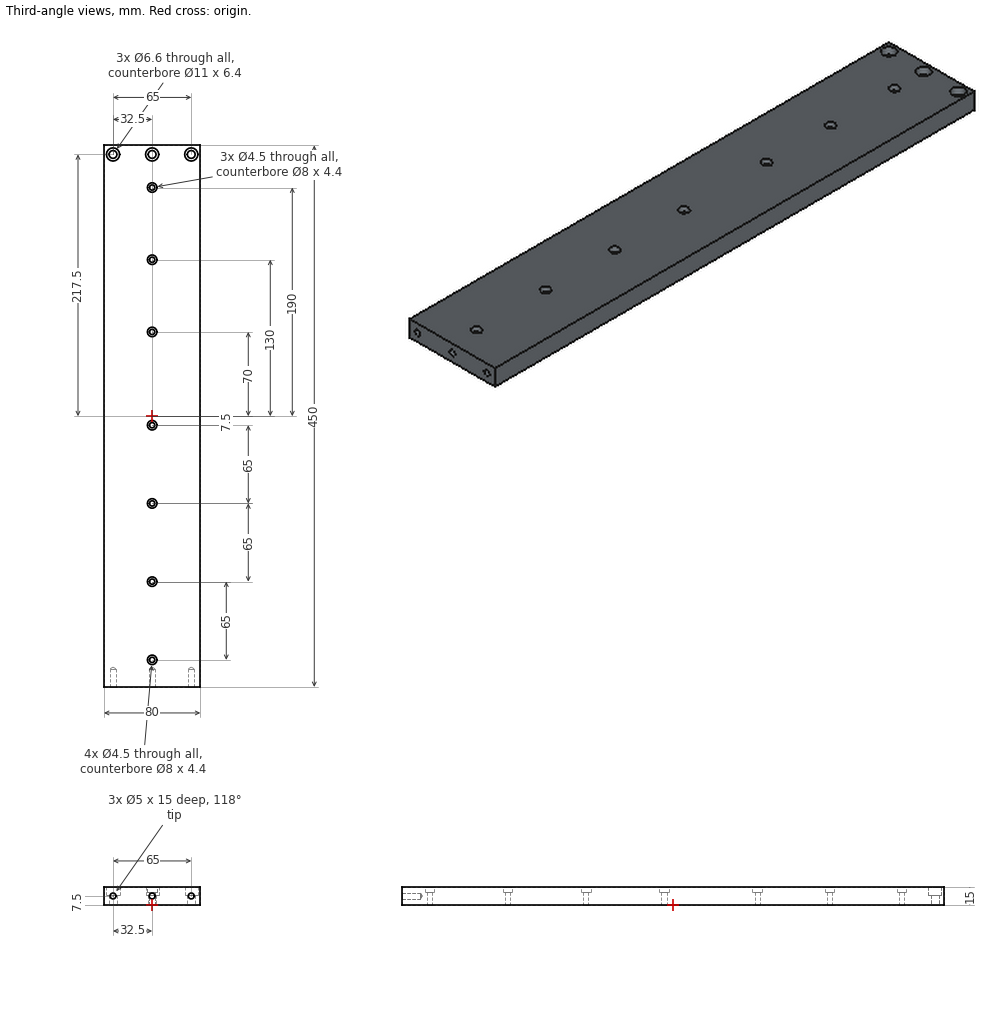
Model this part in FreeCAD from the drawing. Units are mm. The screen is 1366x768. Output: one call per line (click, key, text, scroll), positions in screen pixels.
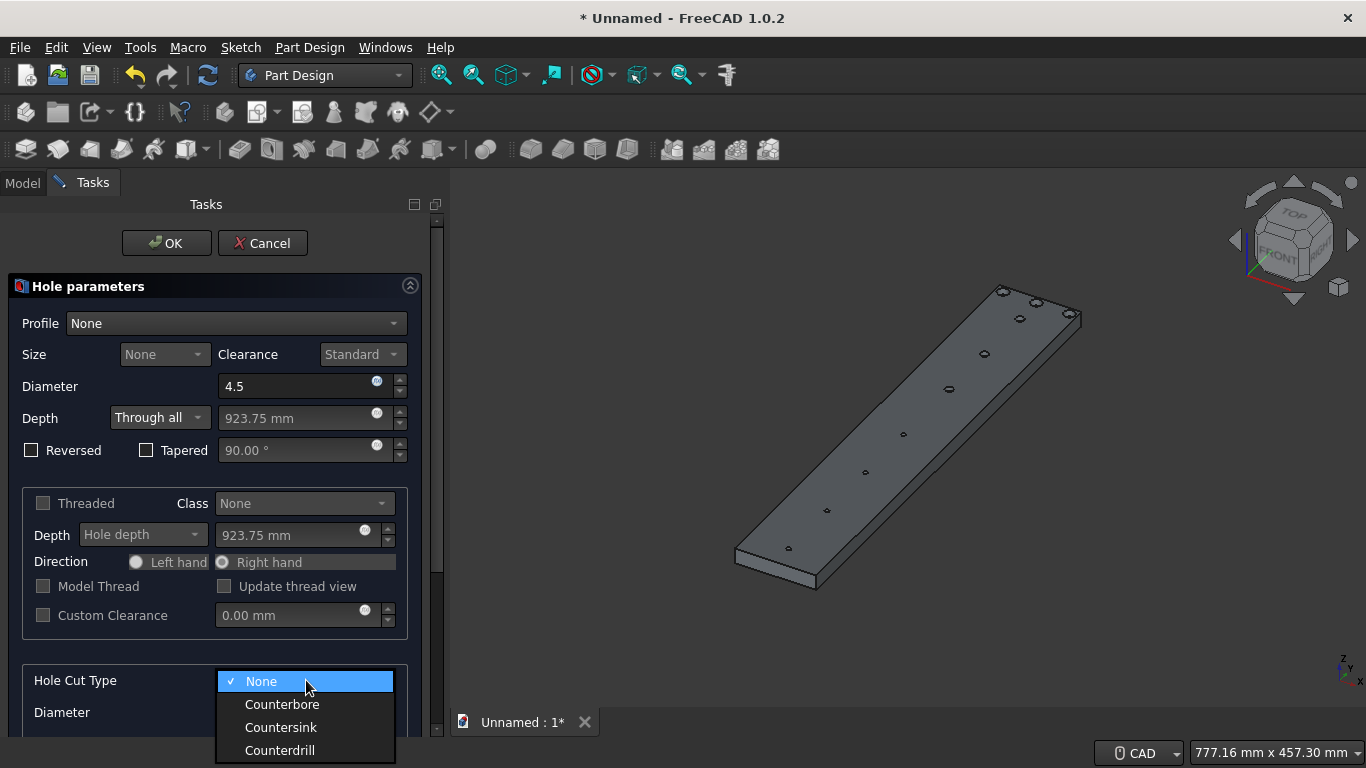
click(304, 704)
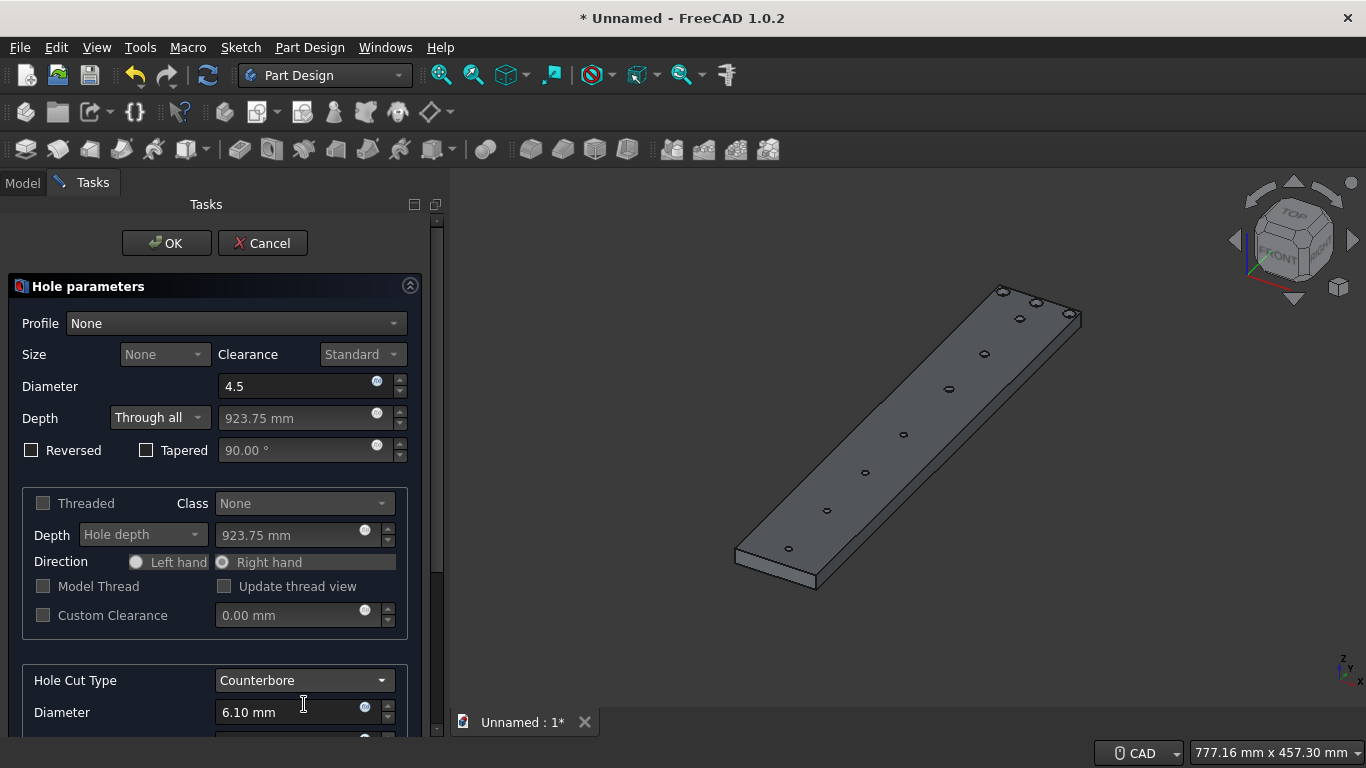
triple_click(298, 712)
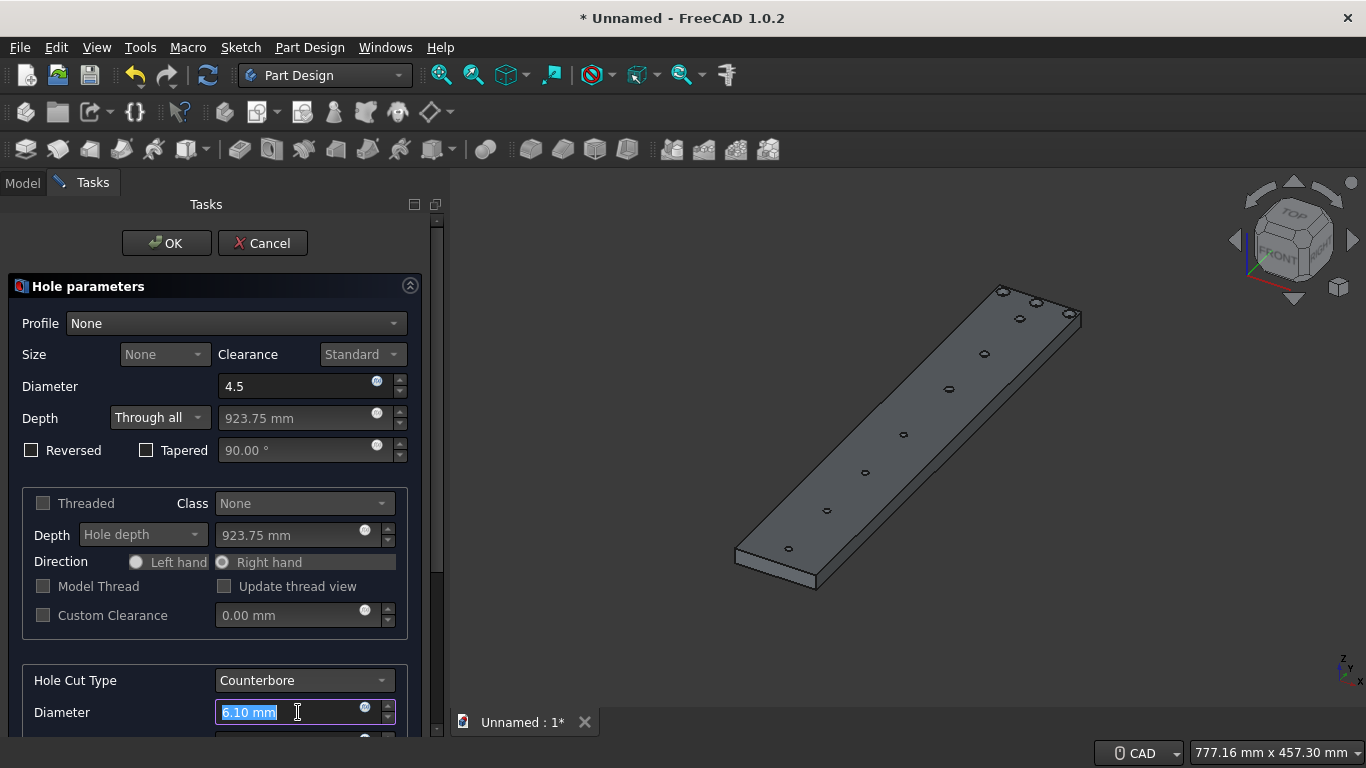
text(8)
key(Tab)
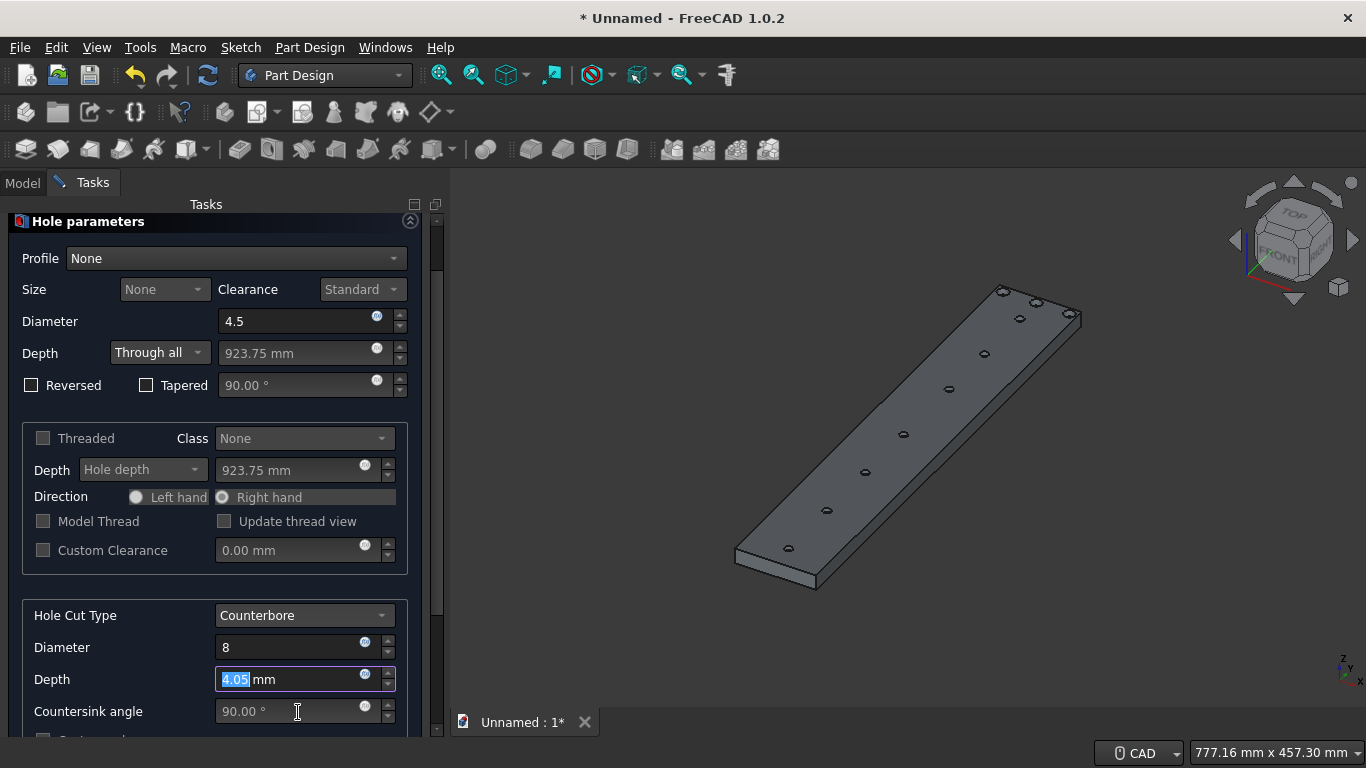
text(4.4)
key(Tab)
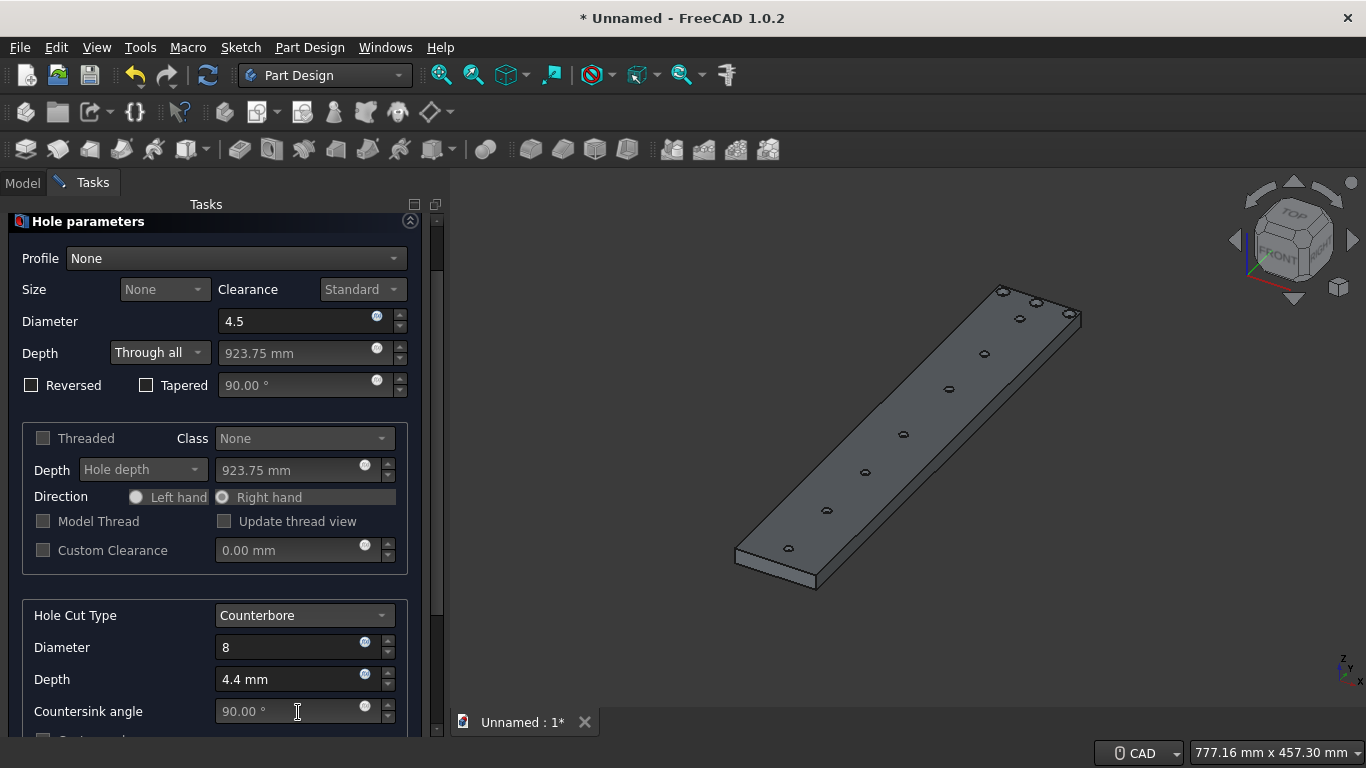
scroll(437, 475, up, 2)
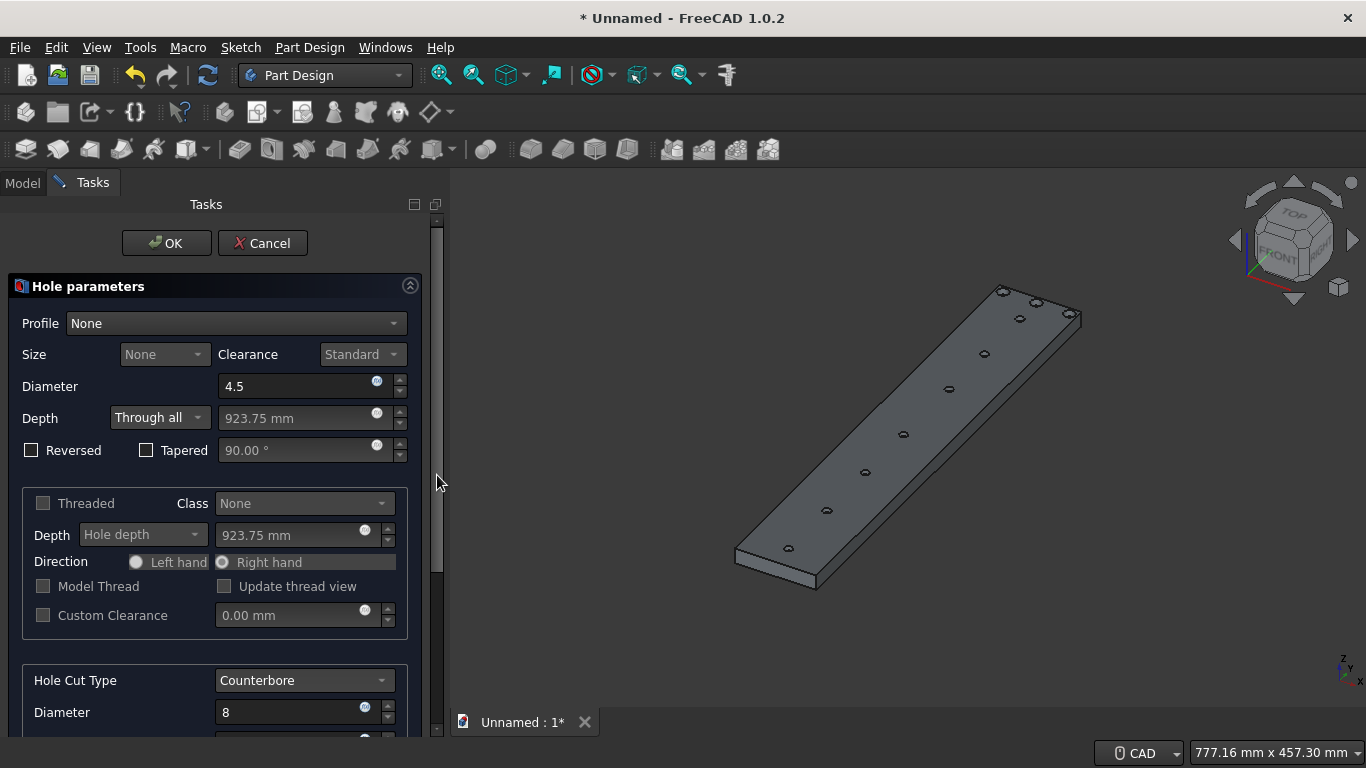
click(167, 243)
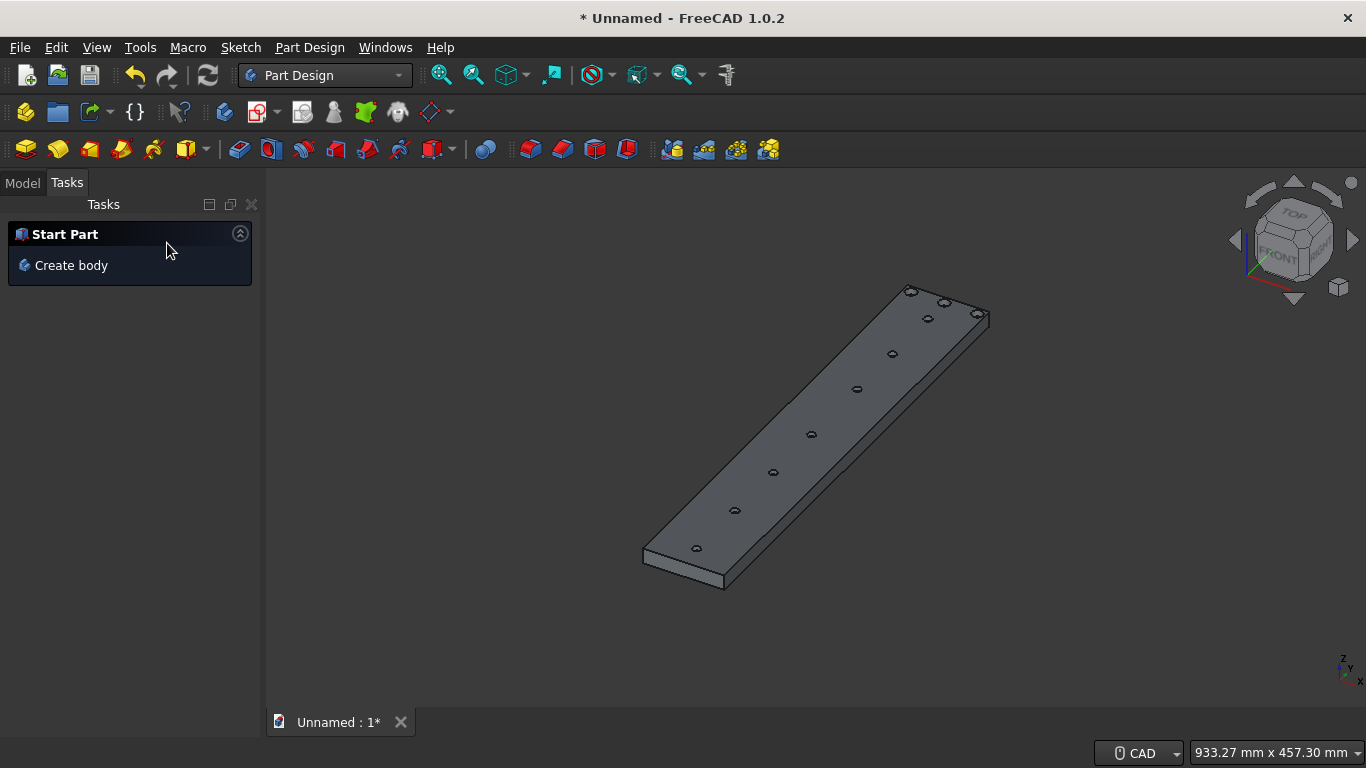
key(0)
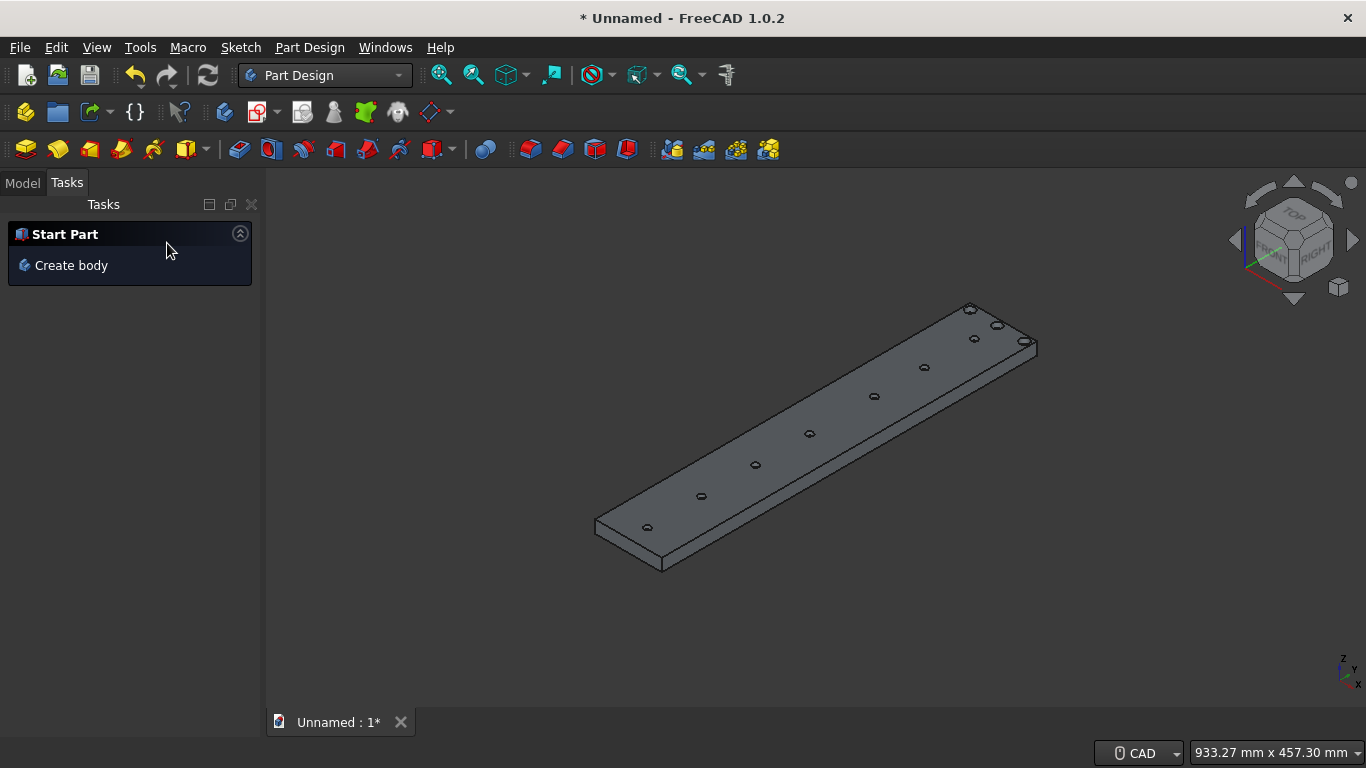
key(1)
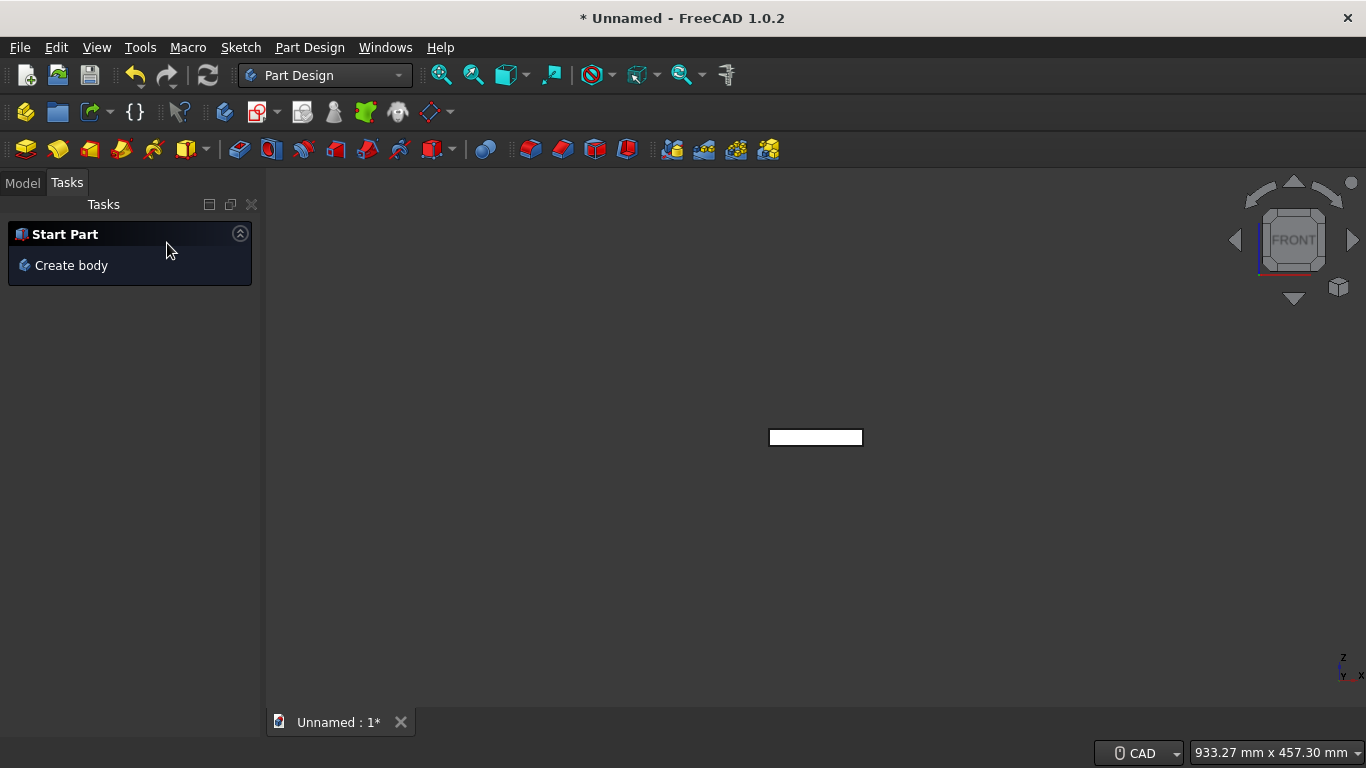
click(442, 76)